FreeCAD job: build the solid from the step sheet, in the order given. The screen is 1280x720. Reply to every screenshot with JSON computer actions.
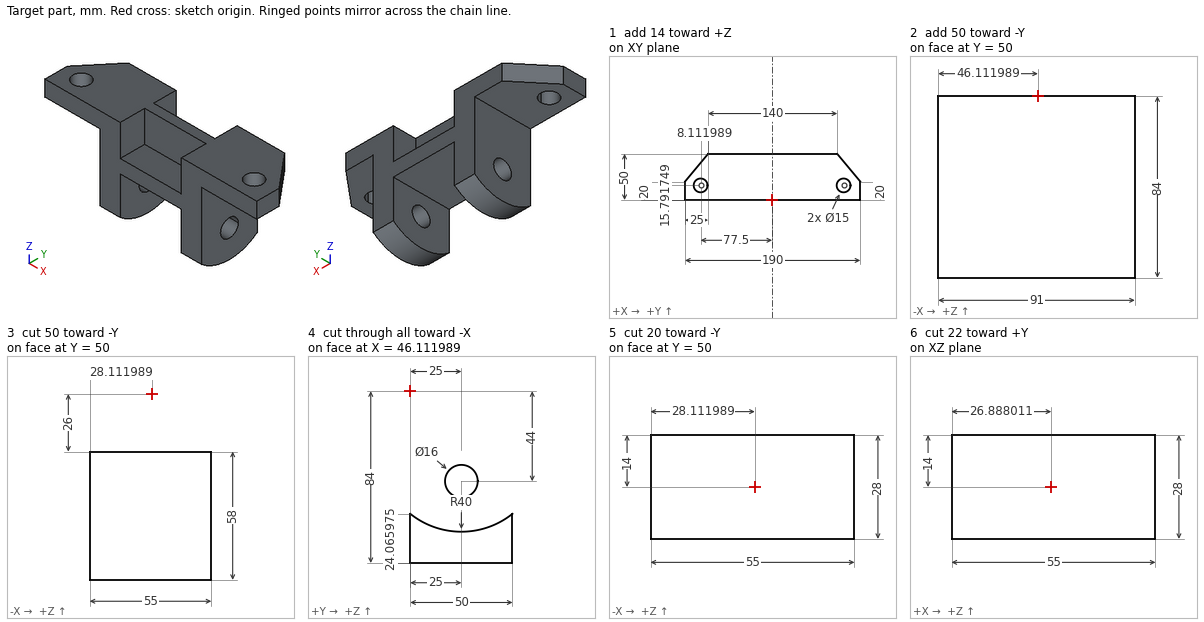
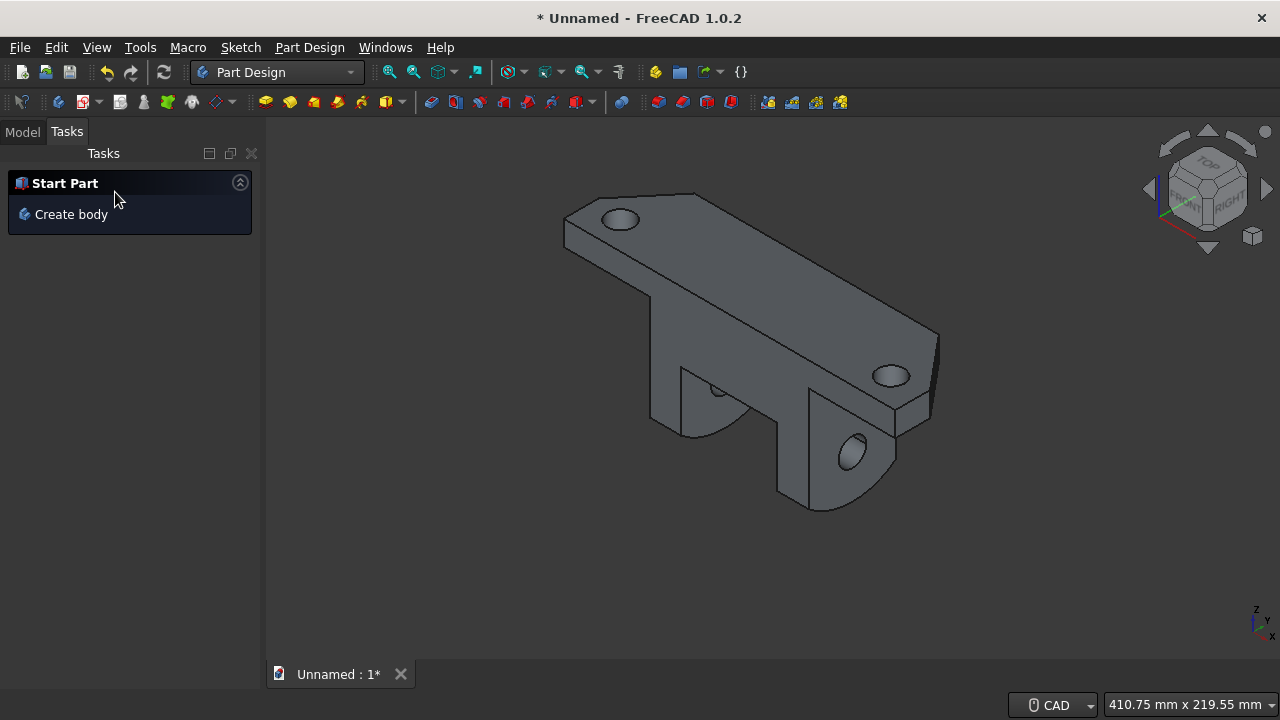
{"action": "key", "text": "4"}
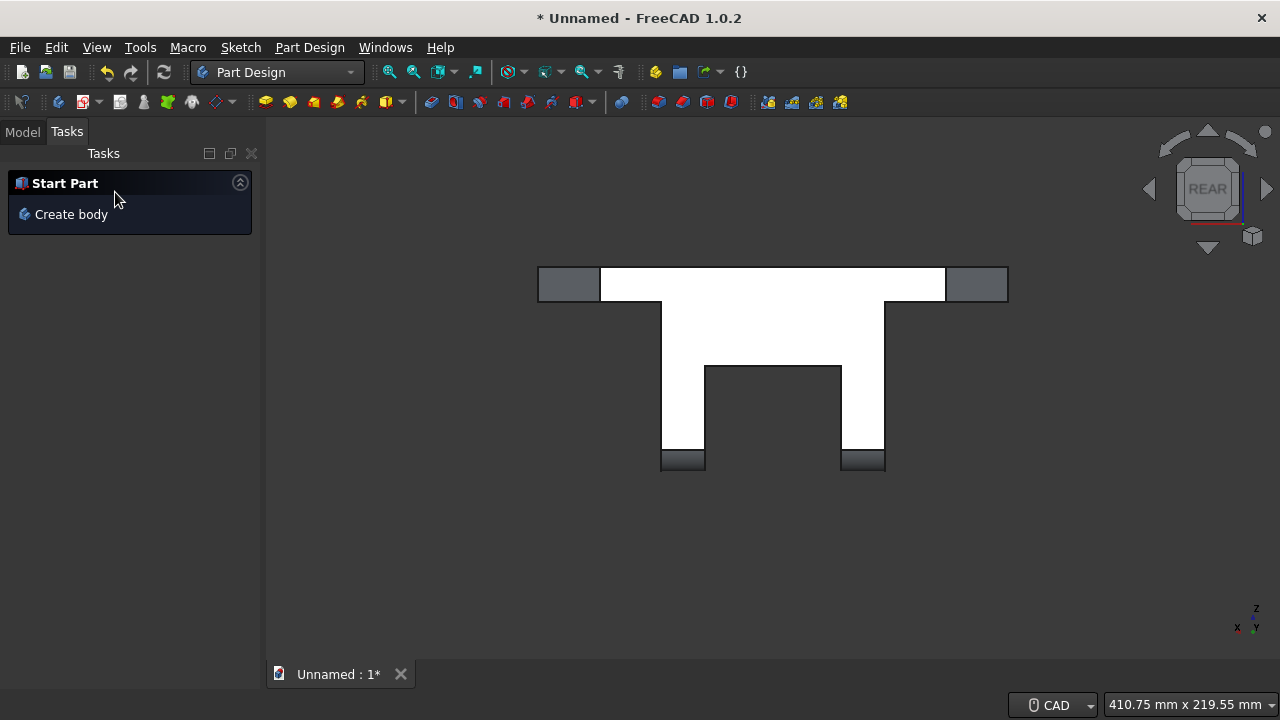
{"action": "left_click", "coordinate": [724, 305]}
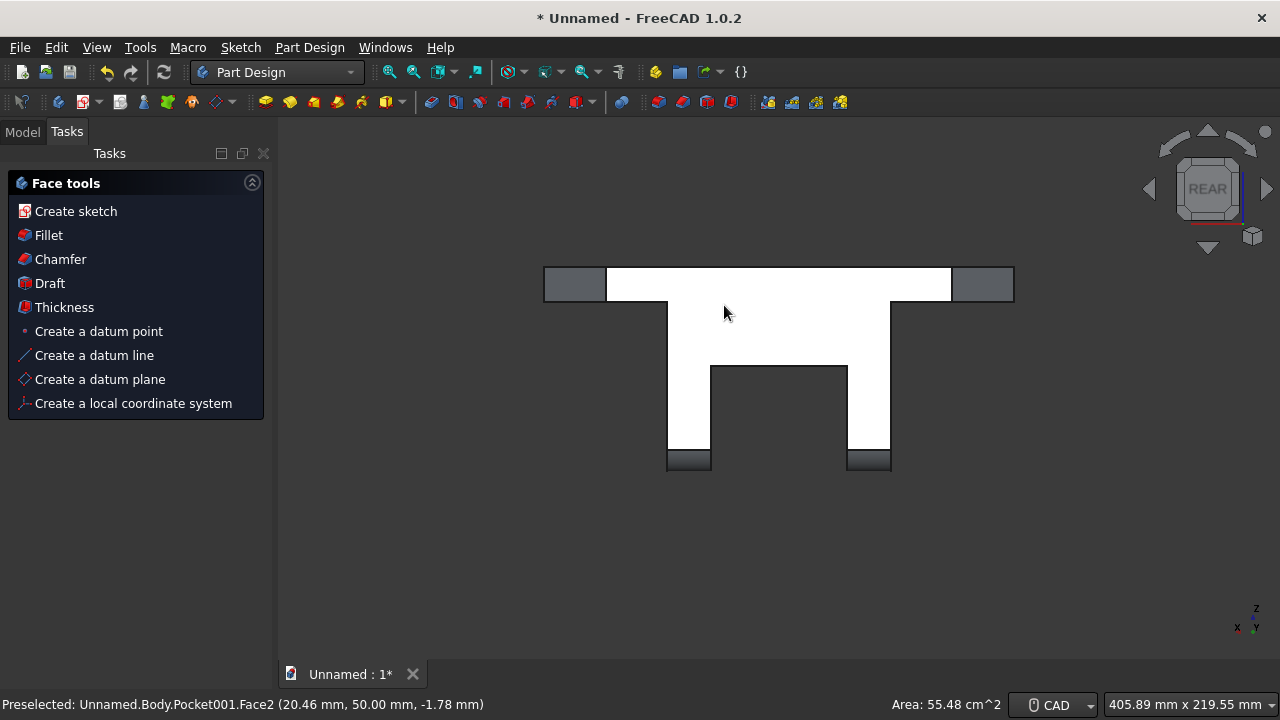
{"action": "left_click", "coordinate": [84, 102]}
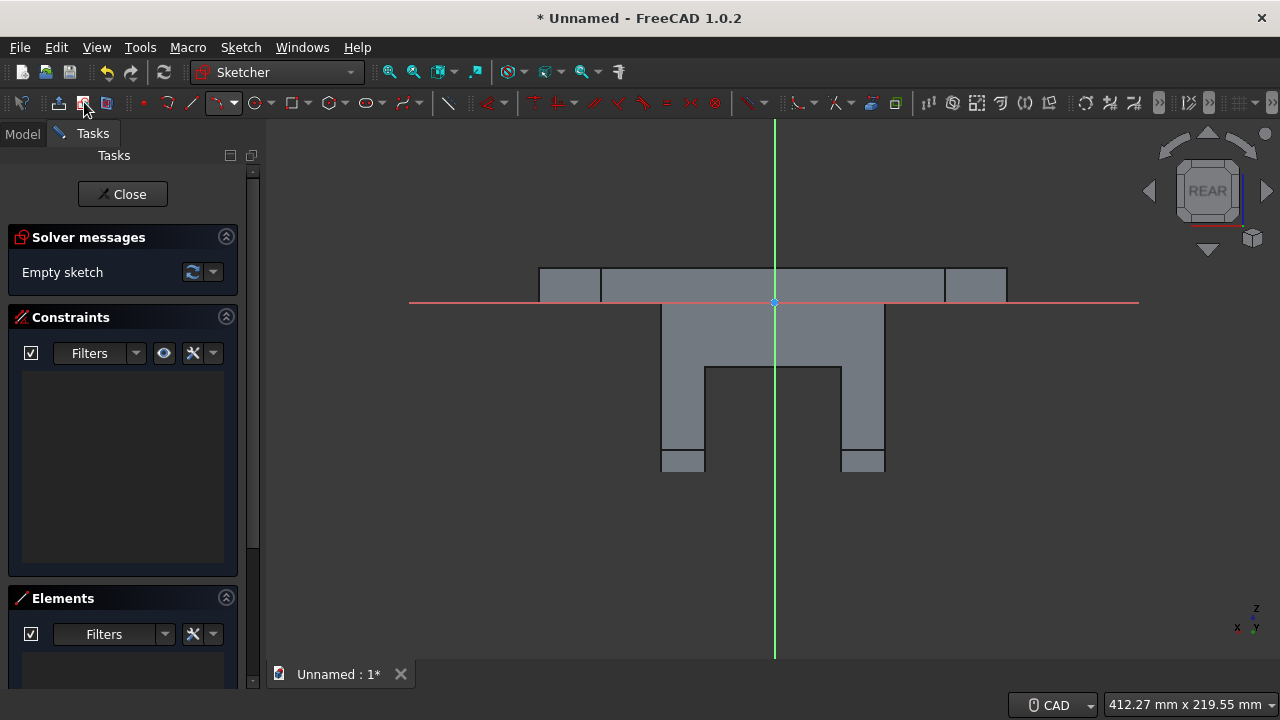
{"action": "scroll", "coordinate": [795, 275], "scroll_direction": "up", "scroll_amount": 7}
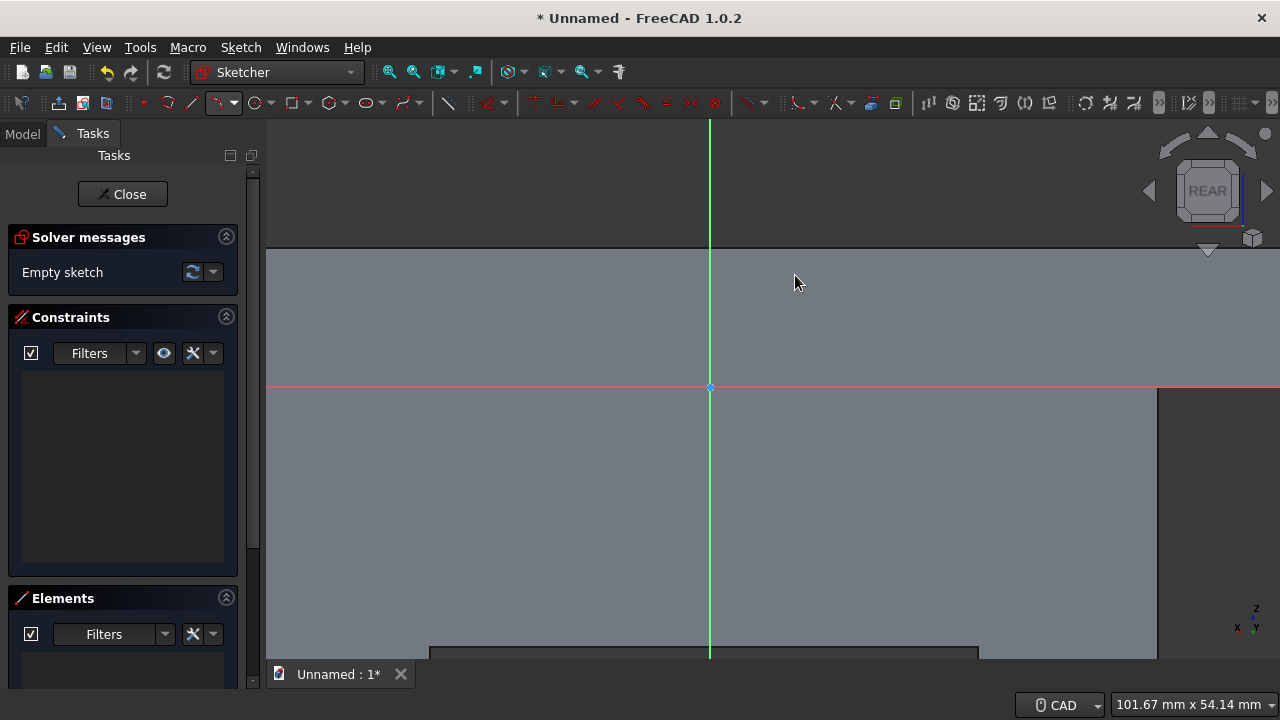
{"action": "left_click", "coordinate": [292, 104]}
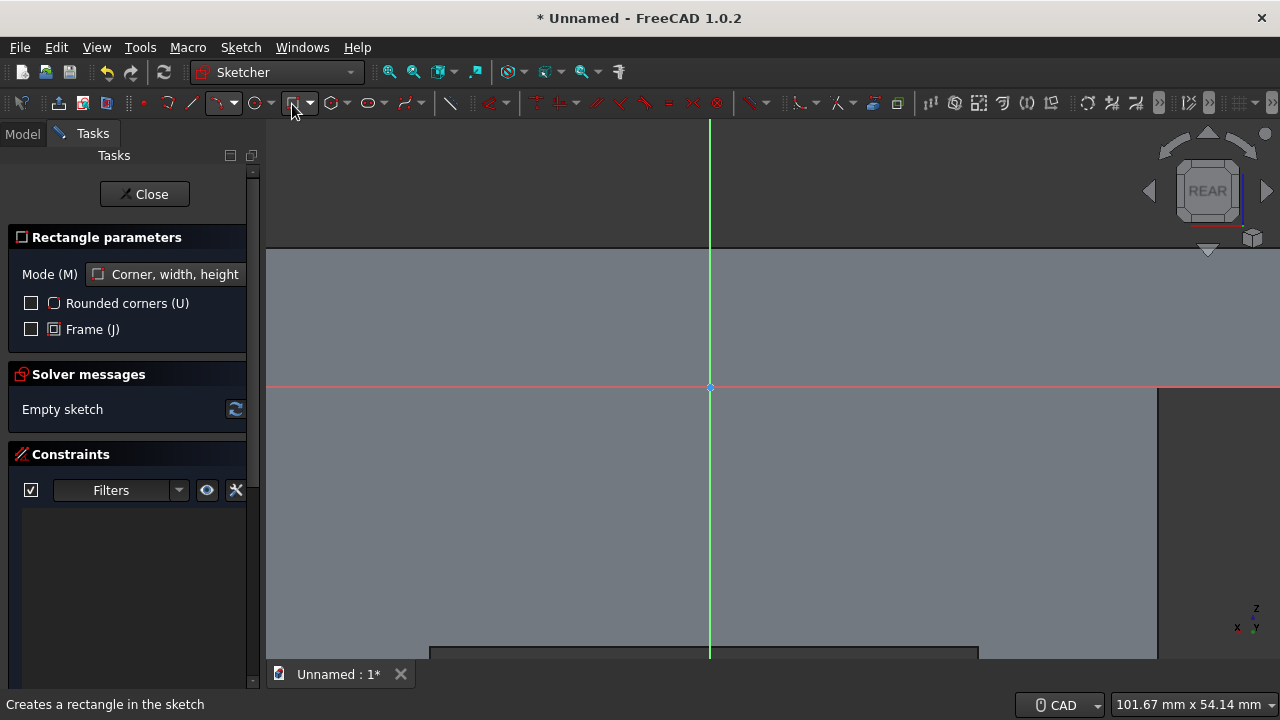
{"action": "left_click", "coordinate": [430, 248]}
{"action": "mouse_move", "coordinate": [978, 527]}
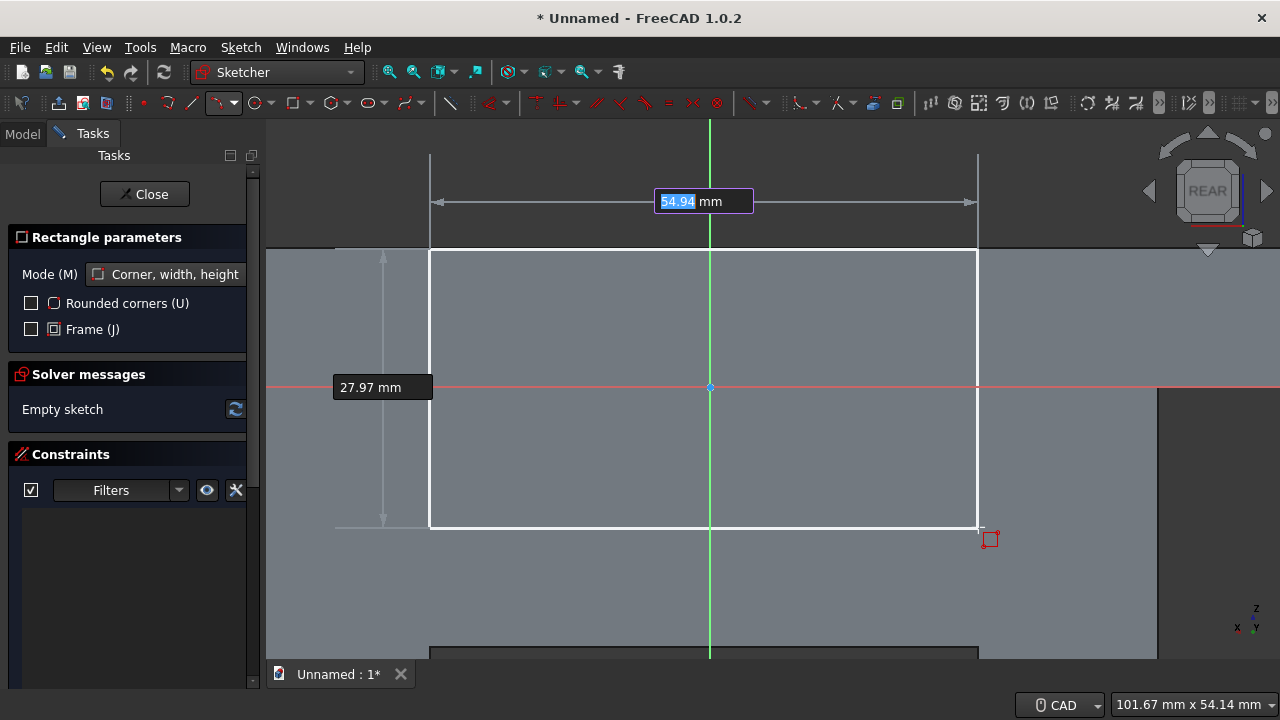
{"action": "type", "text": "55"}
{"action": "key", "text": "Tab"}
{"action": "type", "text": "28"}
{"action": "key", "text": "Return"}
{"action": "key", "text": "Escape"}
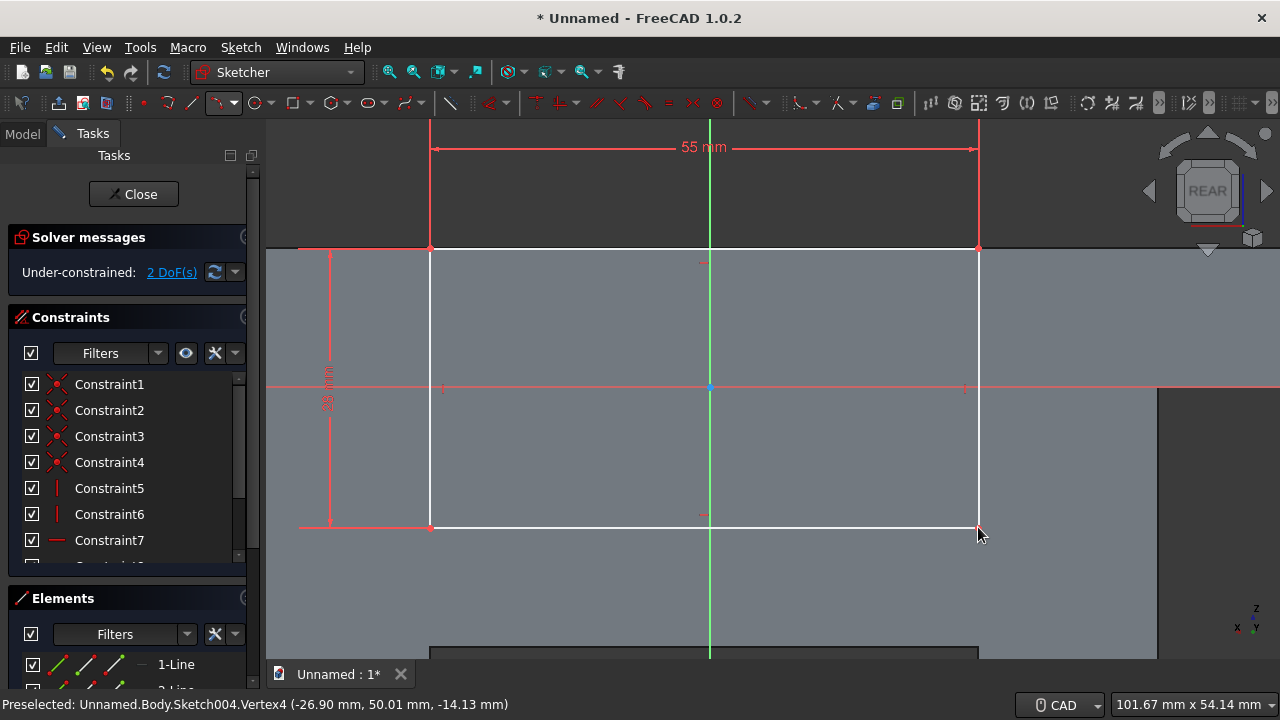
{"action": "left_click", "coordinate": [490, 104]}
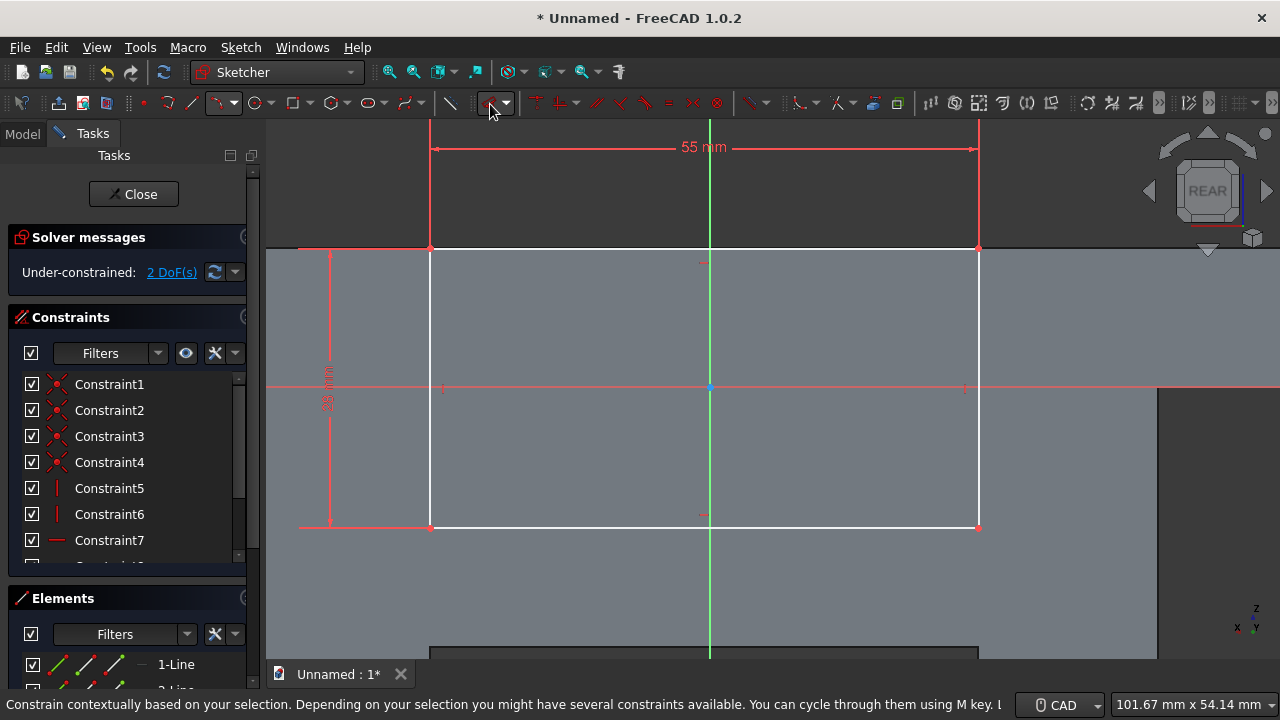
{"action": "left_click", "coordinate": [430, 249]}
{"action": "left_click", "coordinate": [396, 318]}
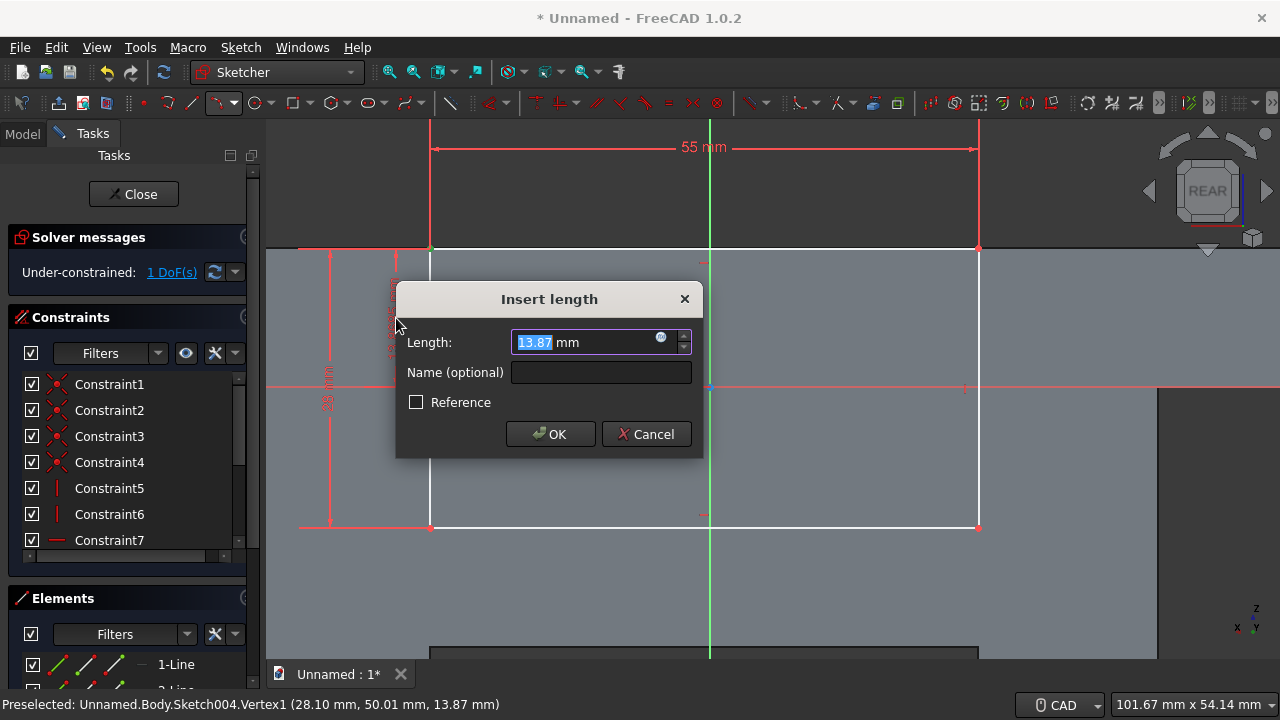
{"action": "type", "text": "14"}
{"action": "key", "text": "Return"}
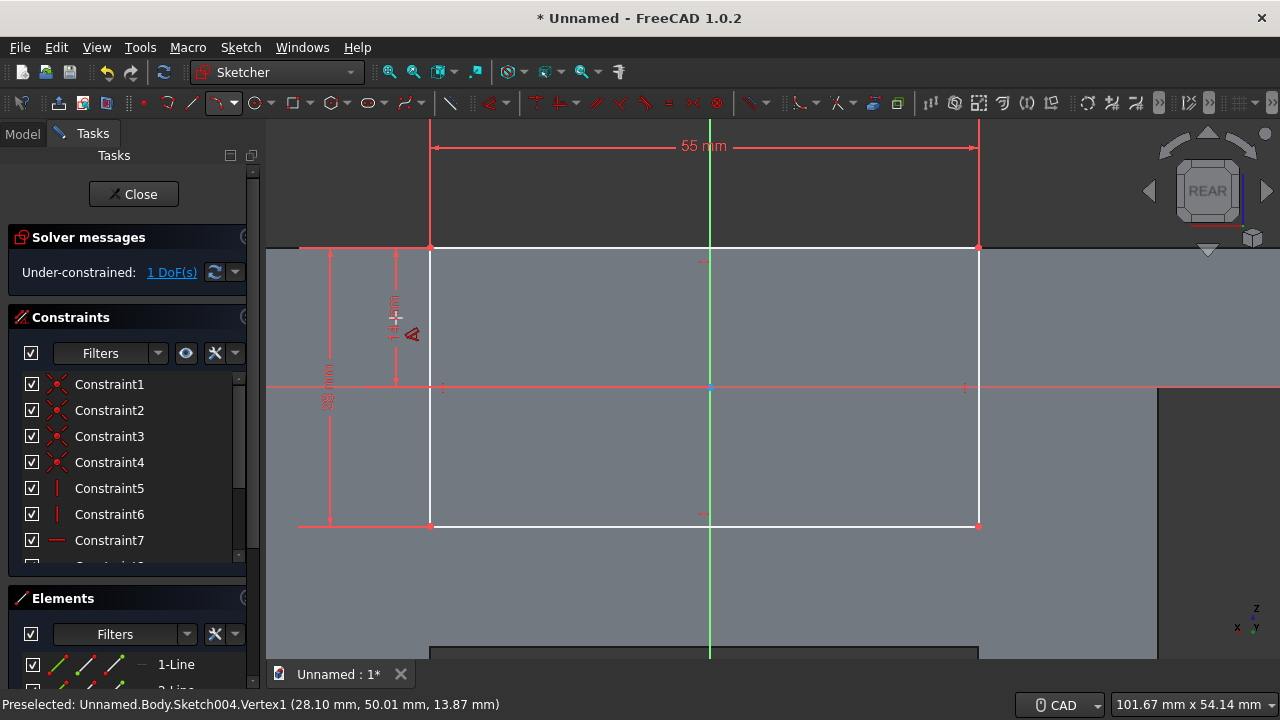
{"action": "left_click", "coordinate": [430, 248]}
{"action": "left_click", "coordinate": [570, 214]}